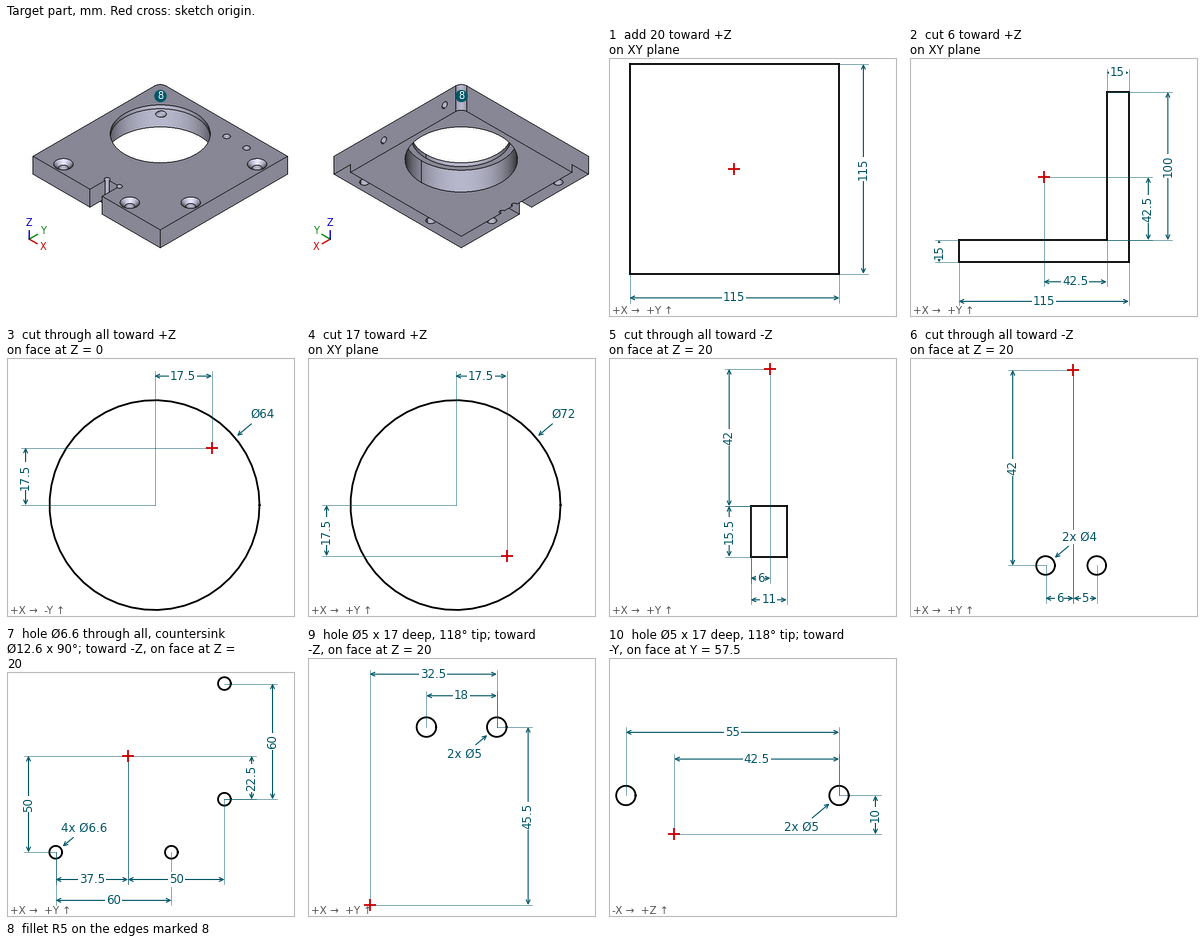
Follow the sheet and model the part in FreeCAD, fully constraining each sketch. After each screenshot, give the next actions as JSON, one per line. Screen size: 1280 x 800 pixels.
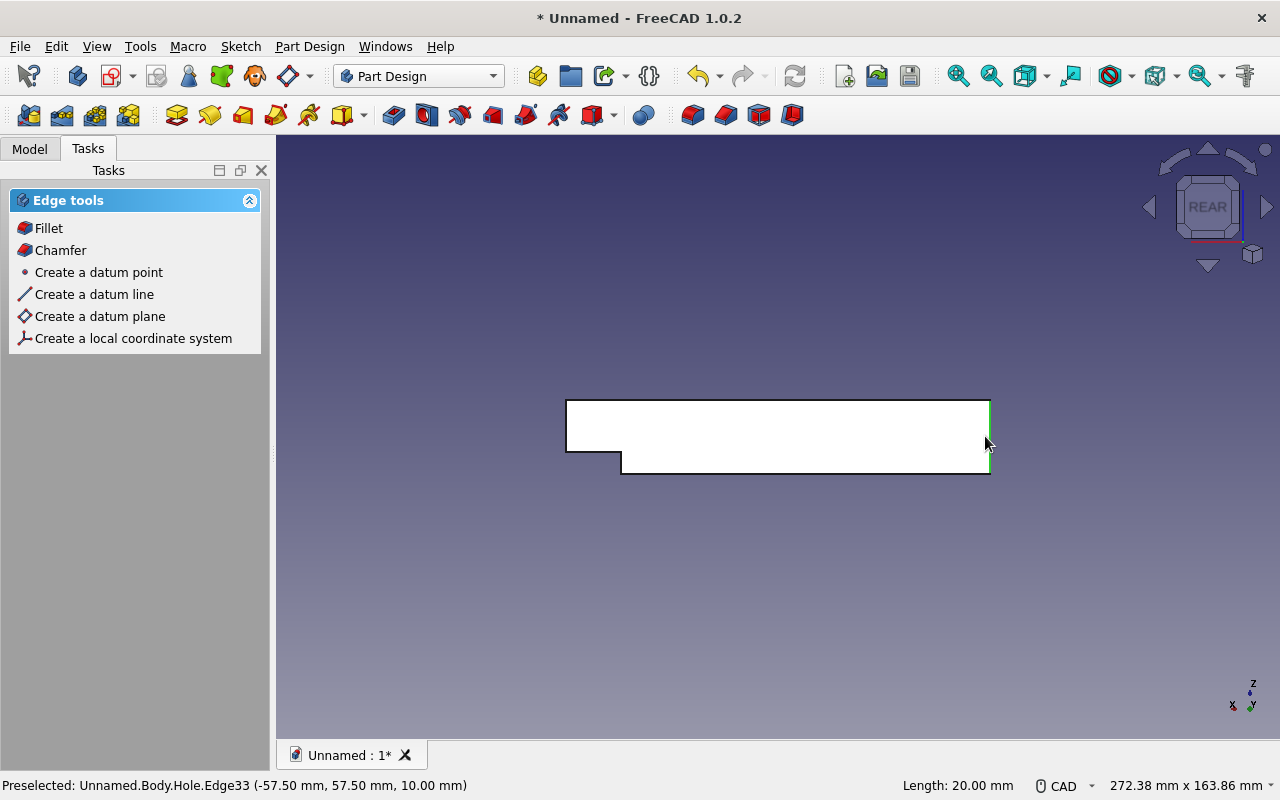
{"action": "left_click", "coordinate": [693, 116]}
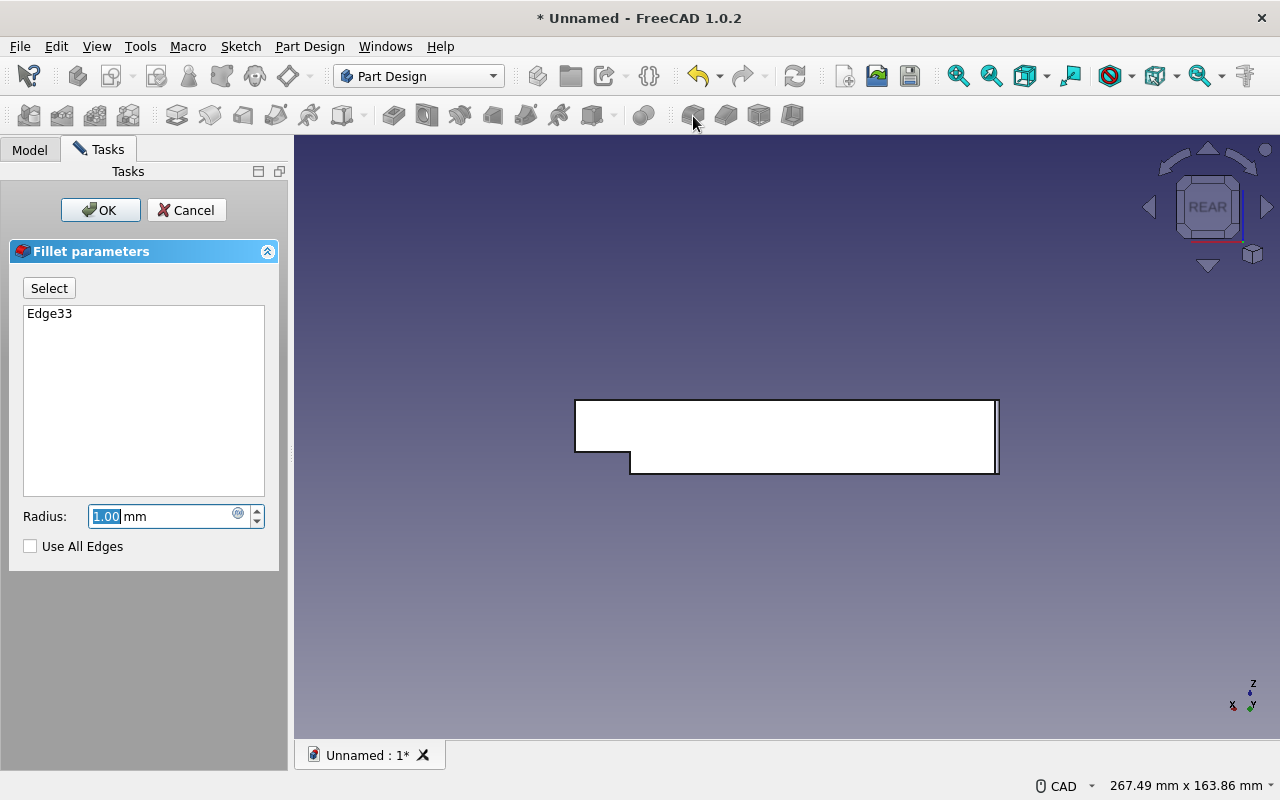
{"action": "type", "text": "5"}
{"action": "key", "text": "Tab"}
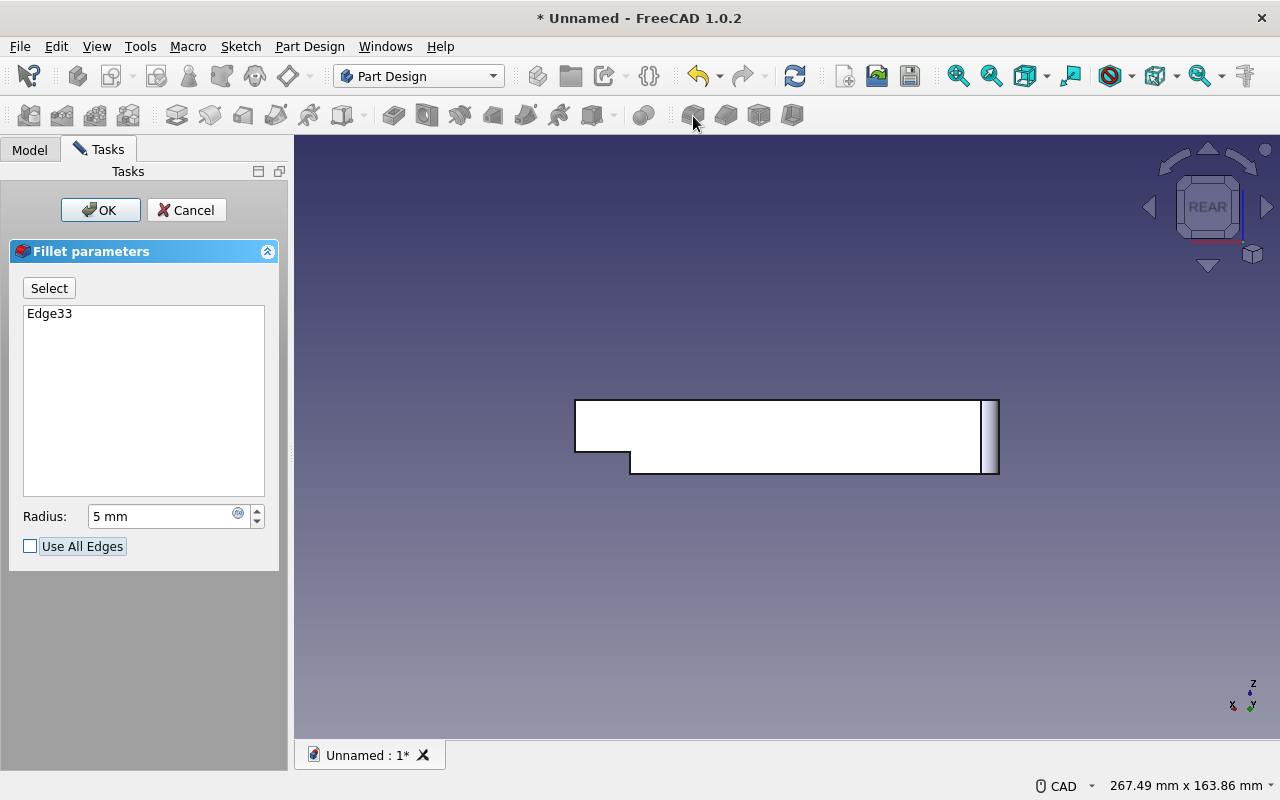
{"action": "left_click", "coordinate": [101, 210]}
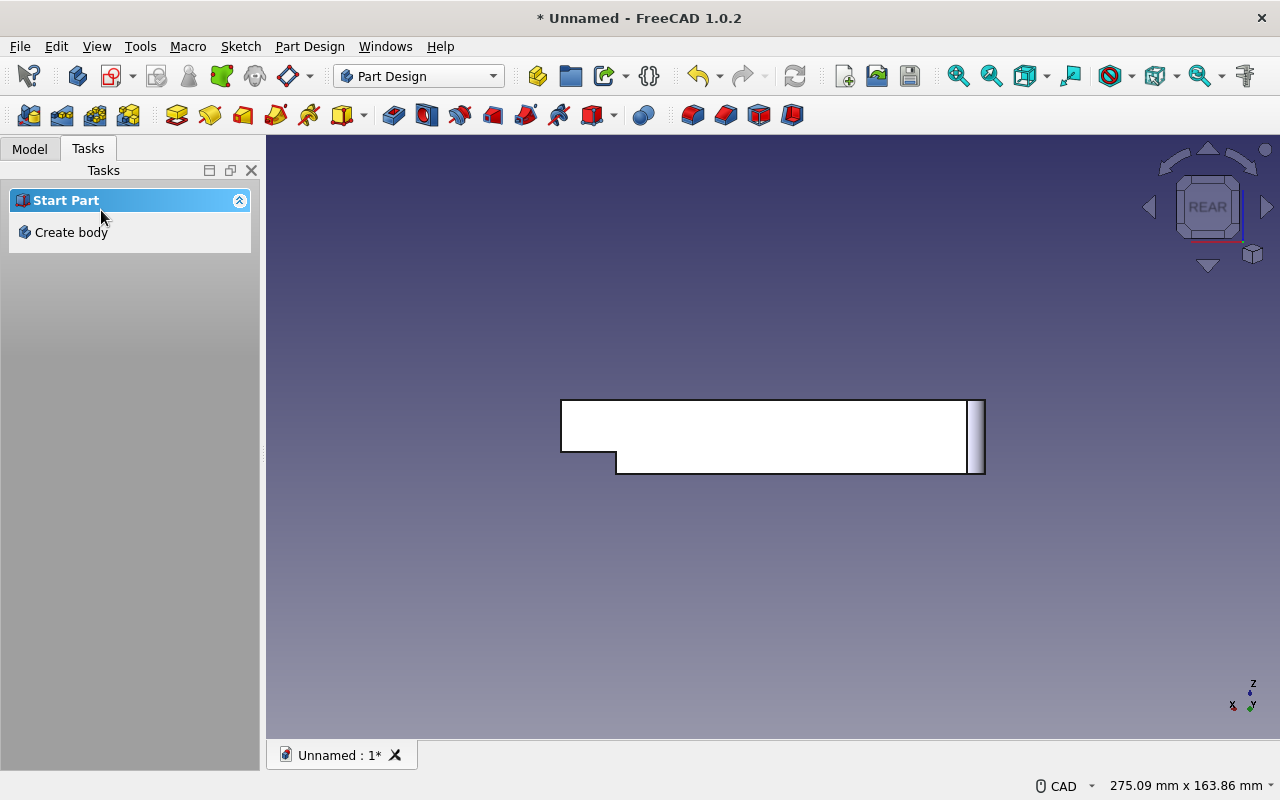
{"action": "key", "text": "v f"}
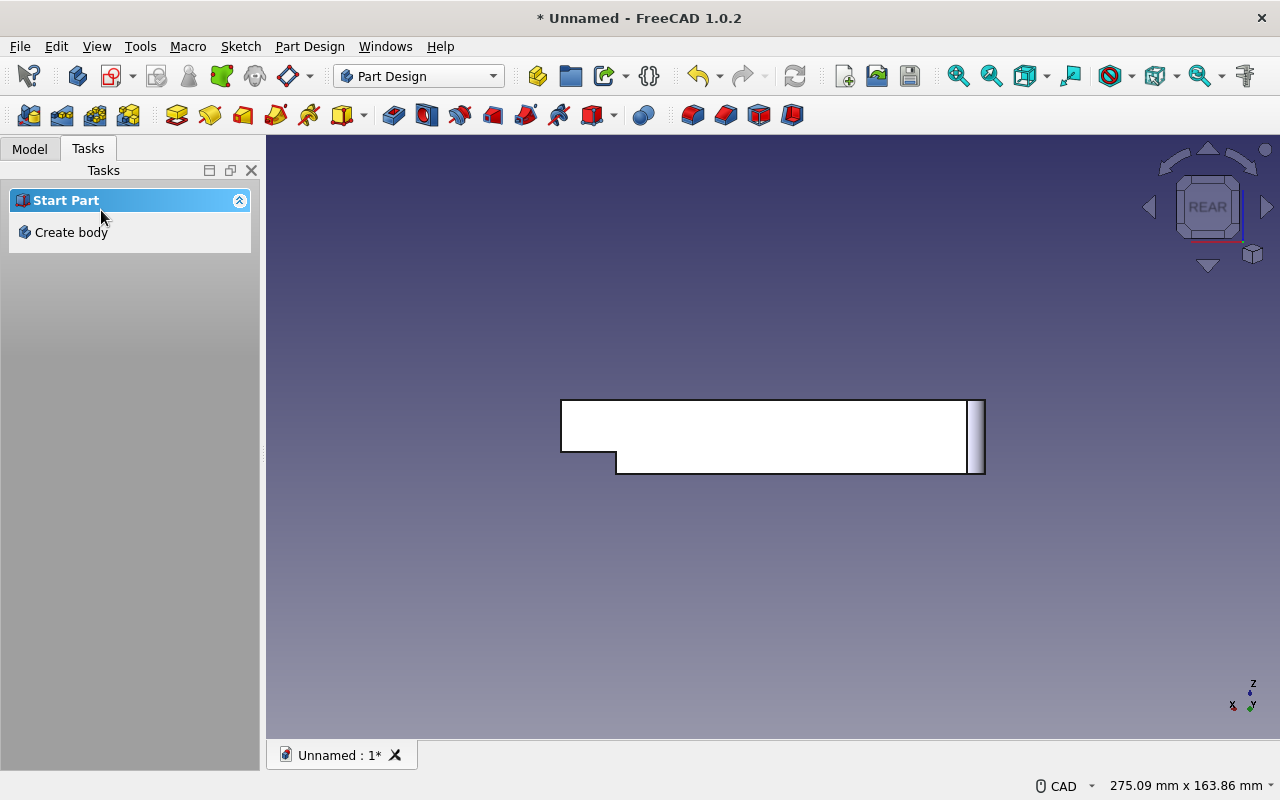
{"action": "key", "text": "0"}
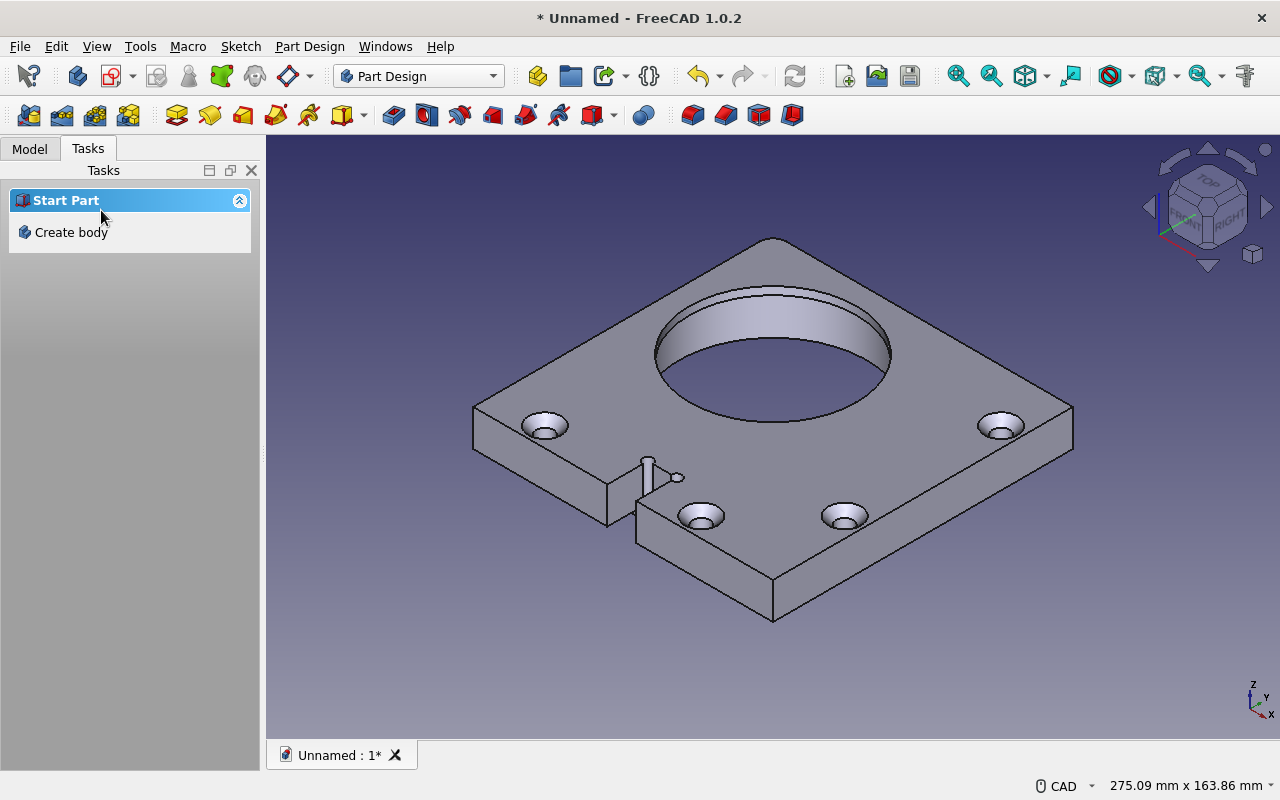
{"action": "left_click", "coordinate": [859, 455]}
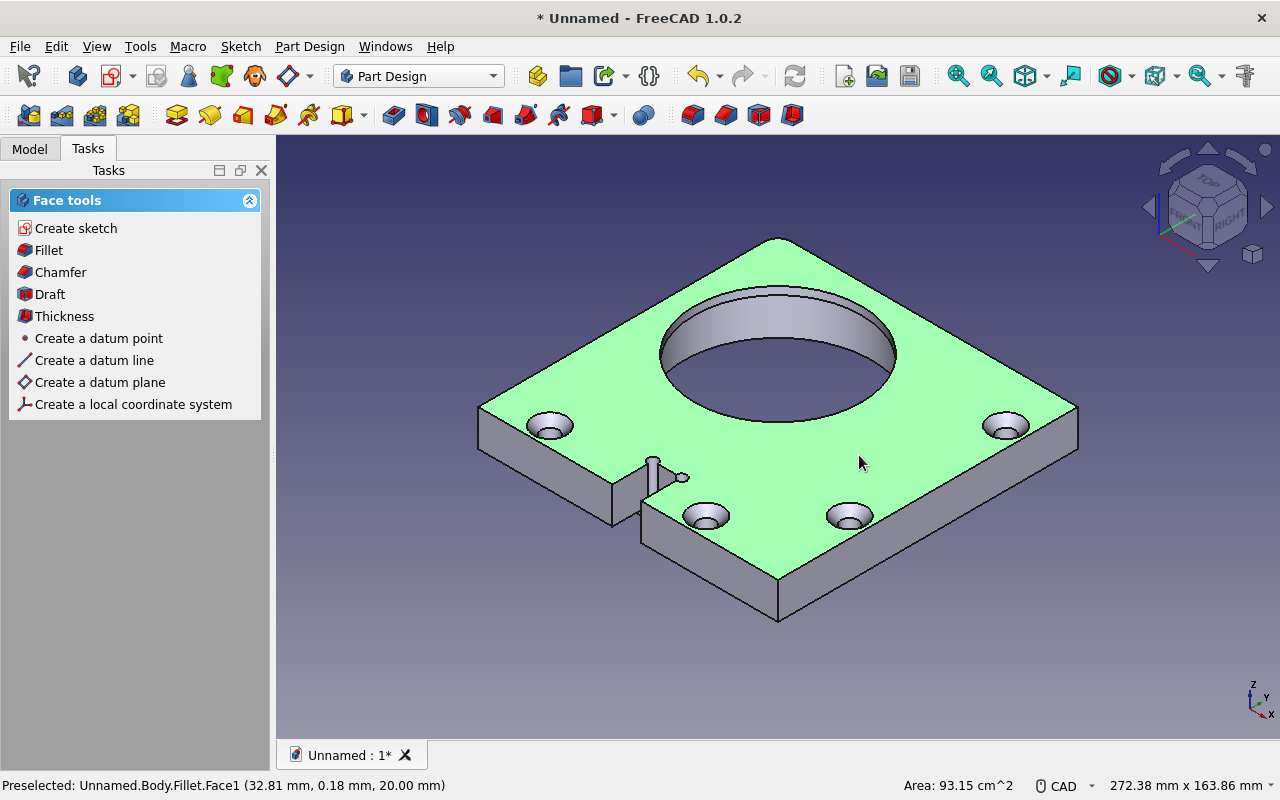
{"action": "left_click", "coordinate": [110, 76]}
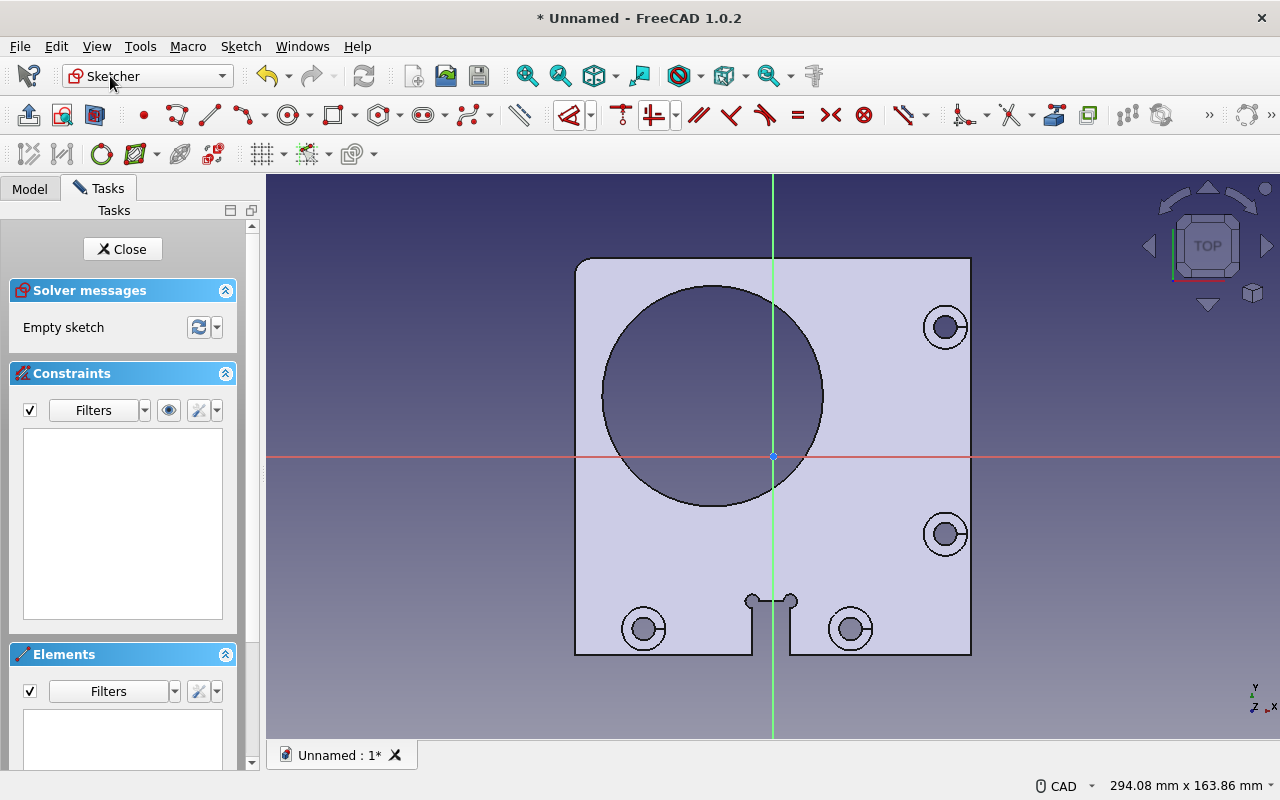
{"action": "scroll", "coordinate": [938, 306], "scroll_direction": "up", "scroll_amount": 4}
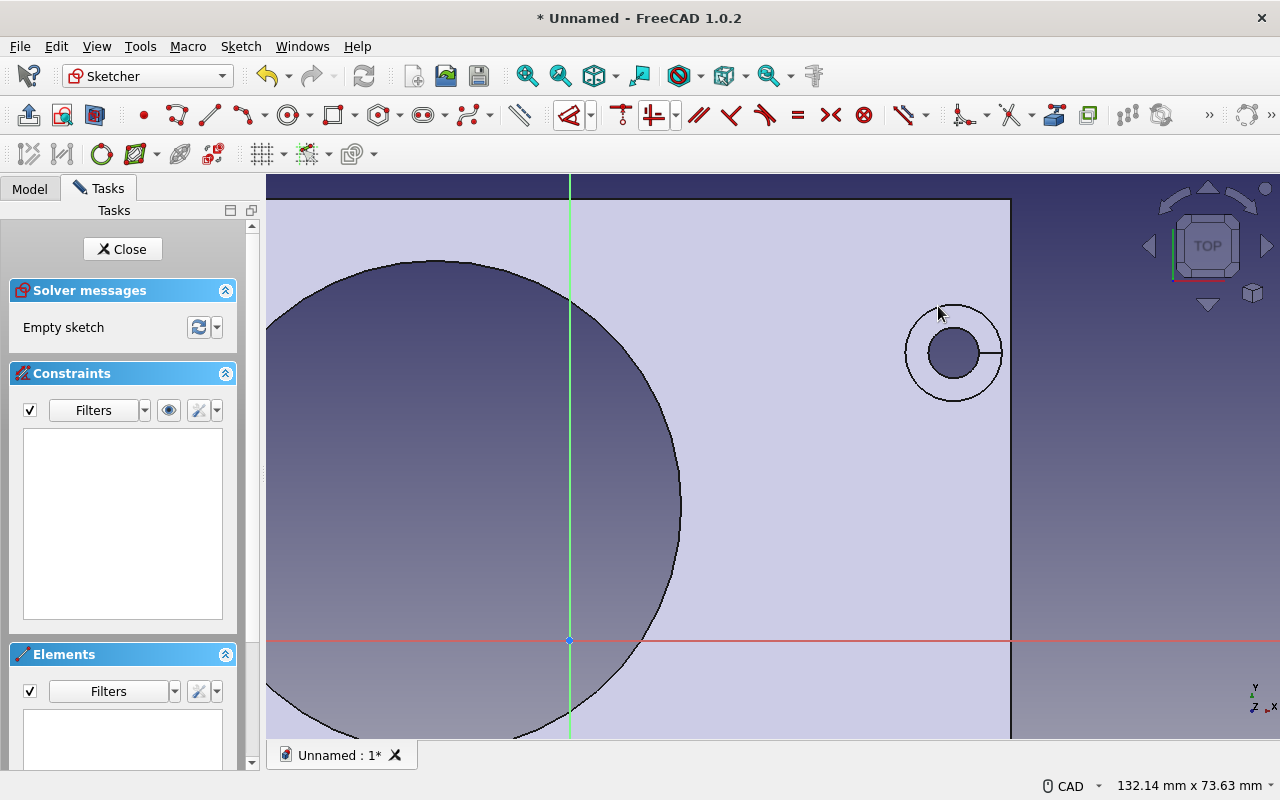
{"action": "key", "text": "g c"}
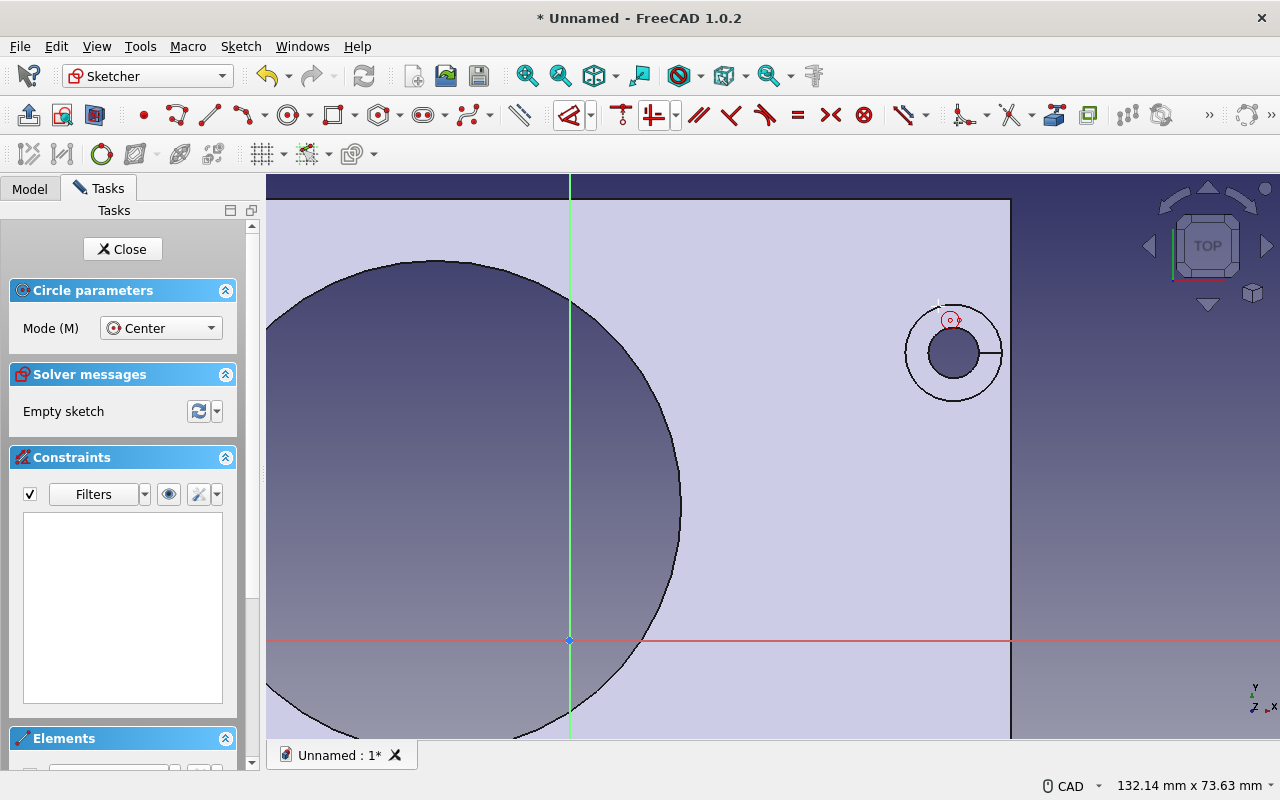
{"action": "left_click", "coordinate": [819, 291]}
{"action": "left_click", "coordinate": [833, 278]}